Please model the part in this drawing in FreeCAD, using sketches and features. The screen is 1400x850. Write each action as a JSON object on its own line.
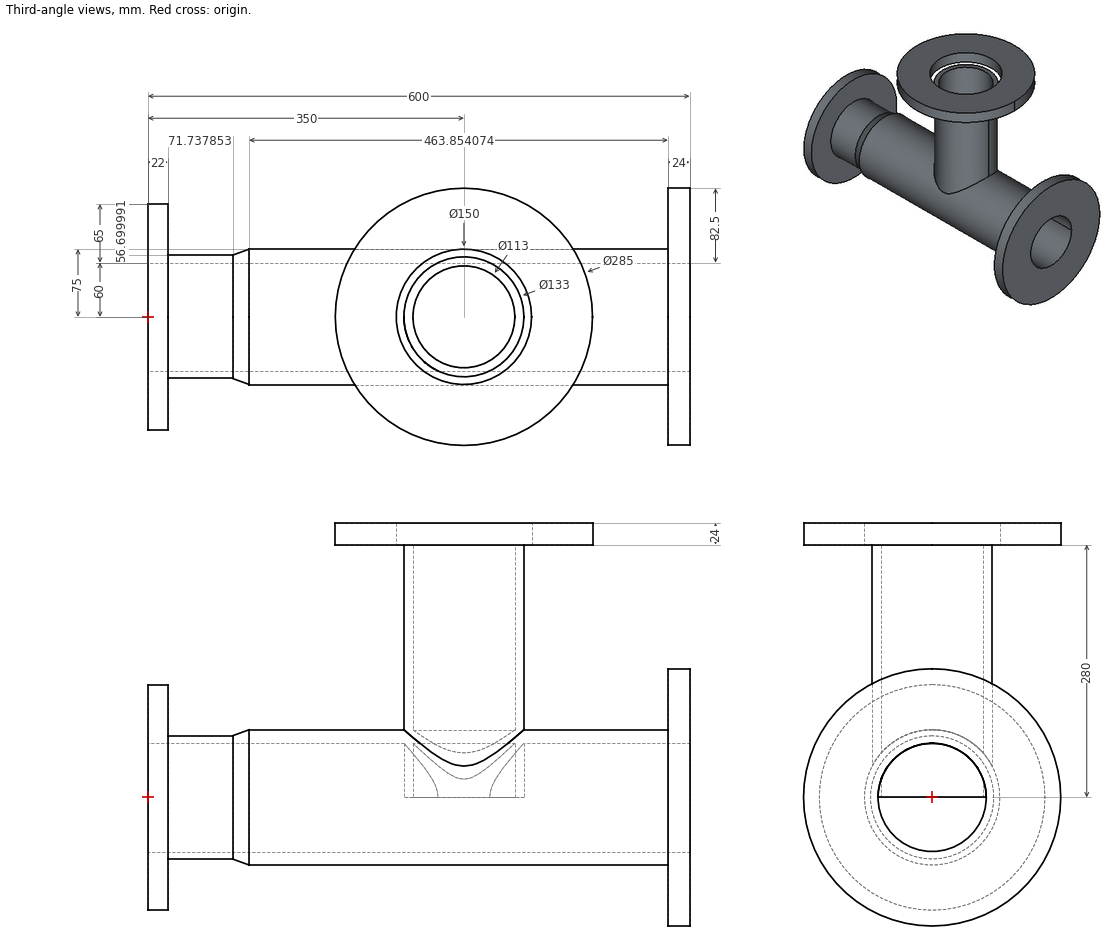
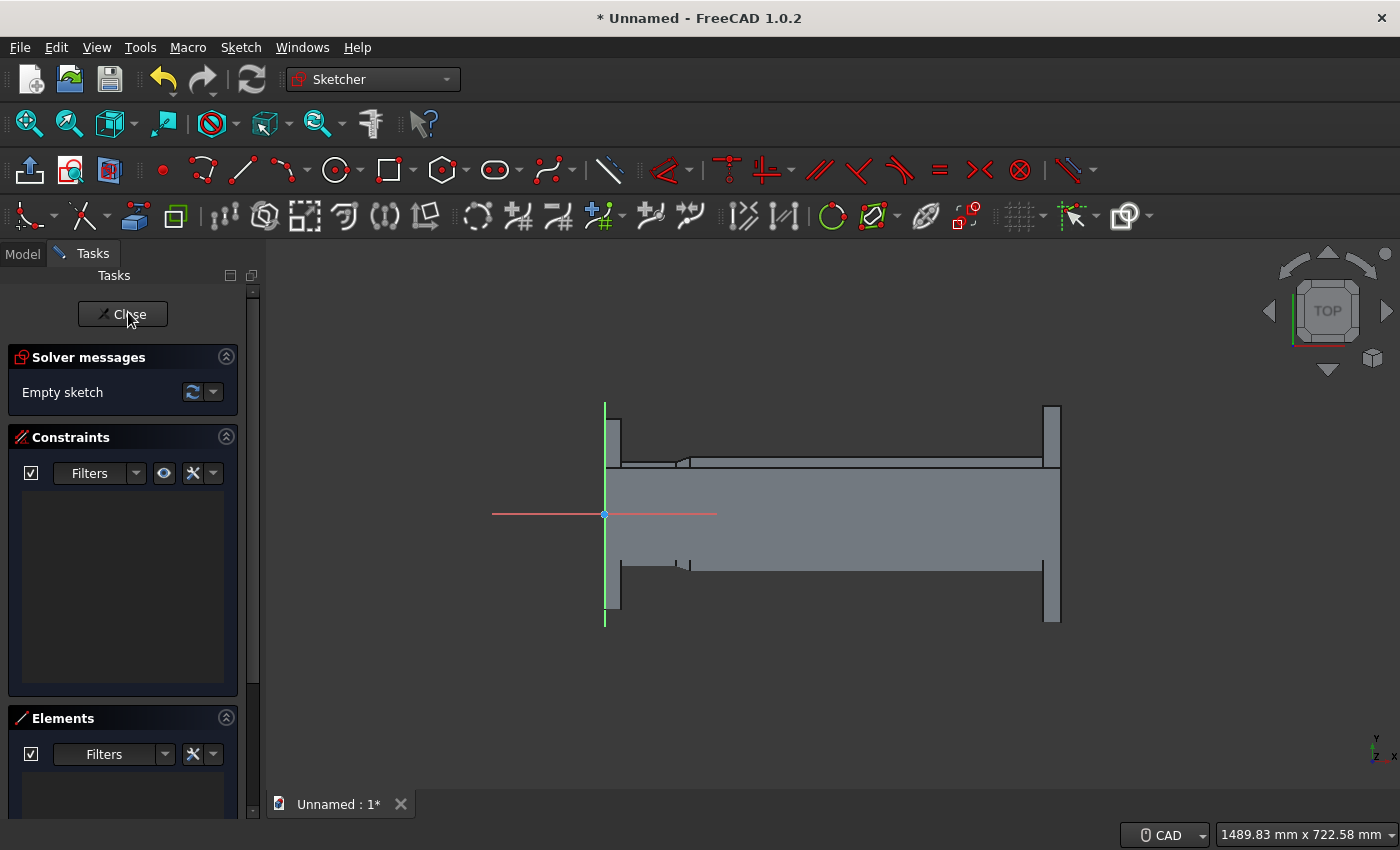
{"action": "scroll", "coordinate": [917, 514], "scroll_direction": "up", "scroll_amount": 6}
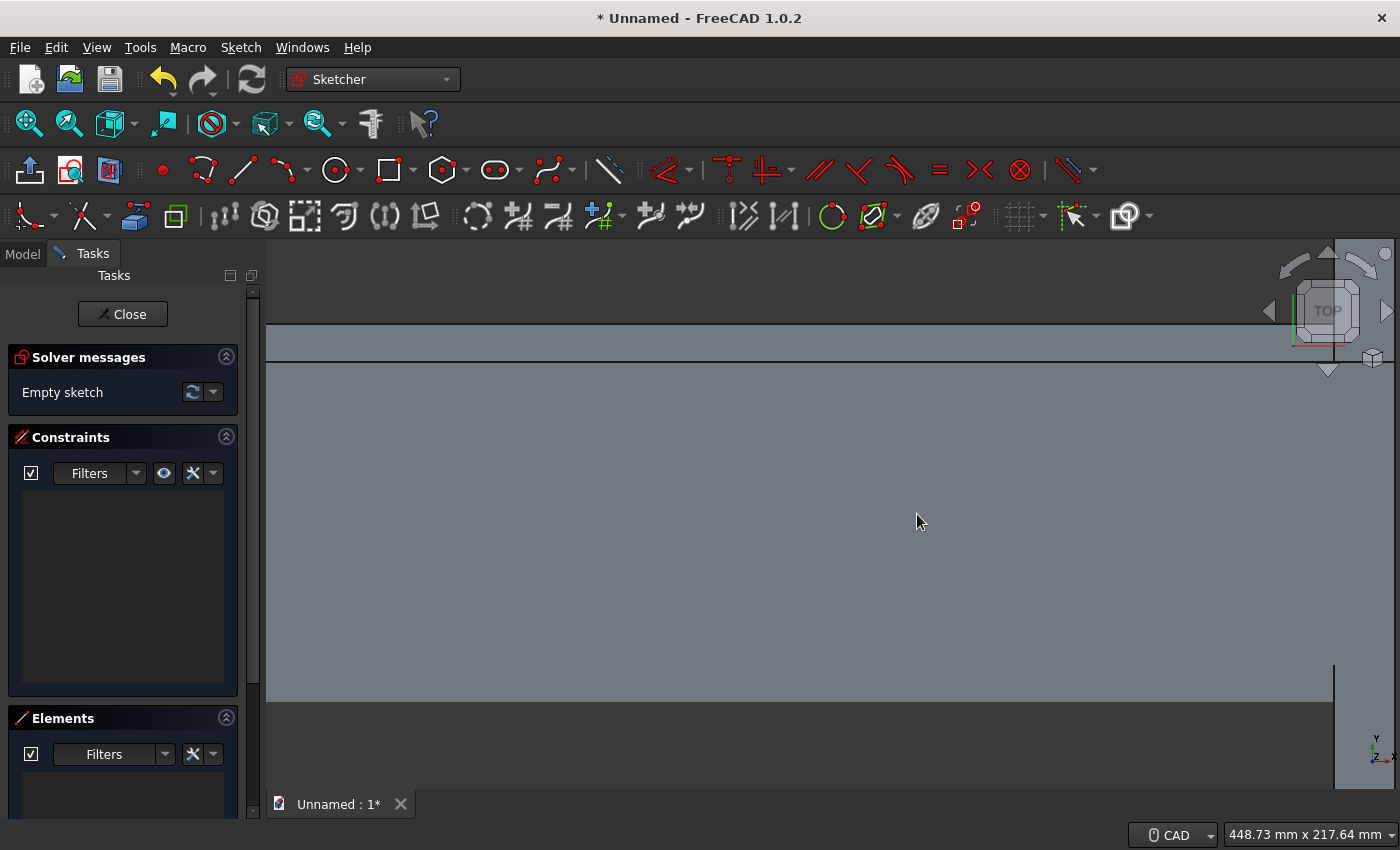
{"action": "key", "text": "g c"}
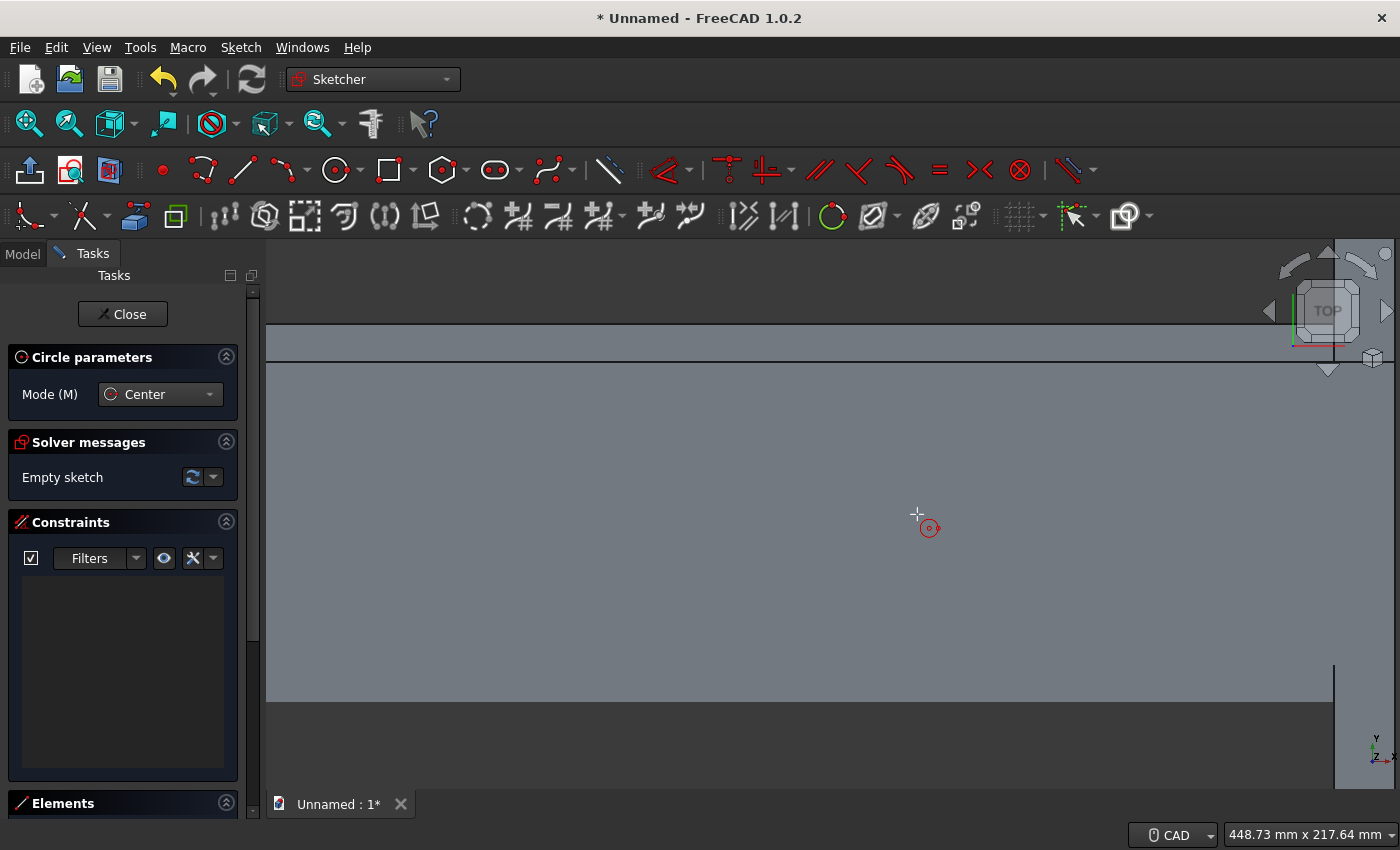
{"action": "left_click", "coordinate": [763, 513]}
{"action": "mouse_move", "coordinate": [882, 394]}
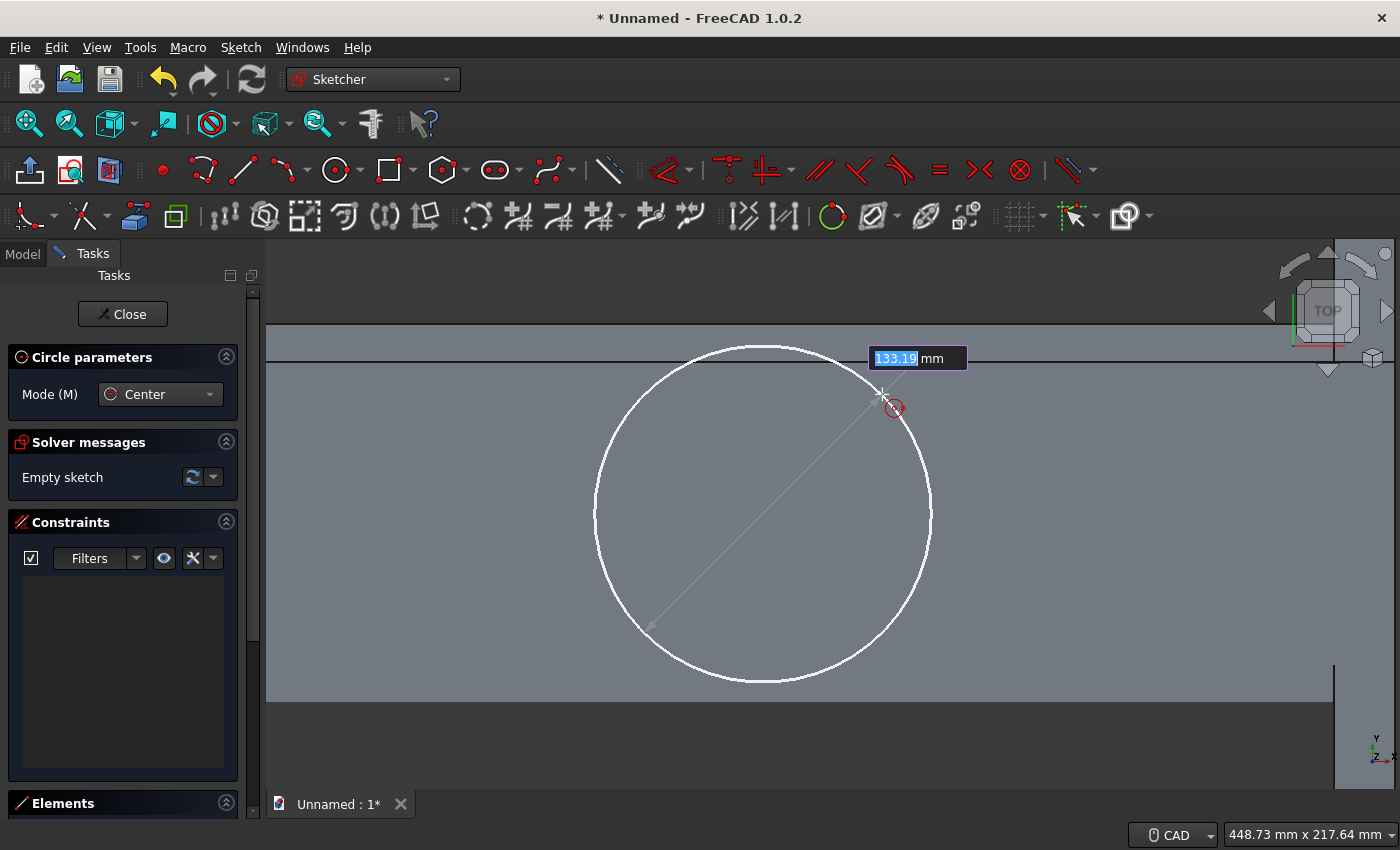
{"action": "type", "text": "133"}
{"action": "key", "text": "Return"}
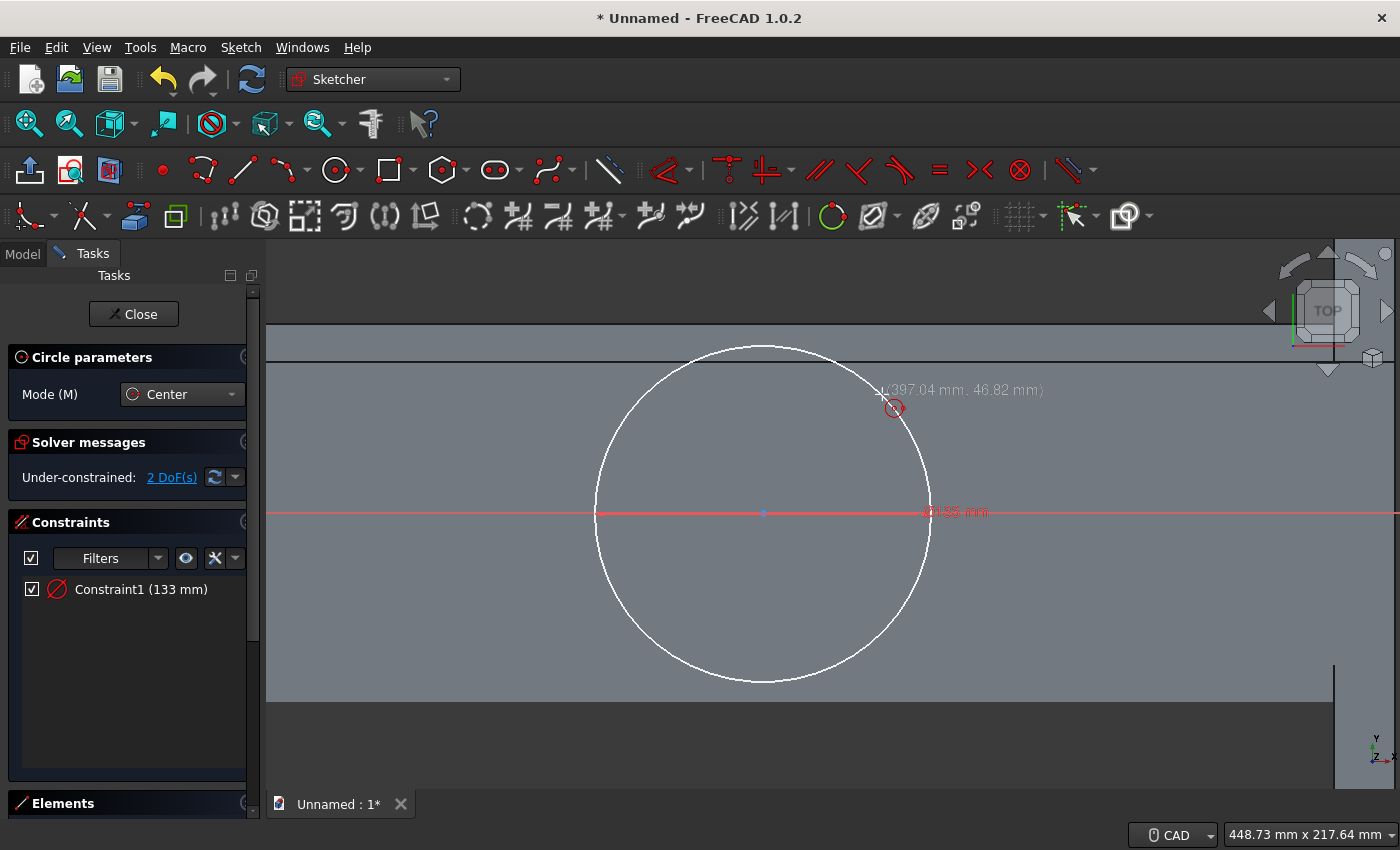
{"action": "left_click", "coordinate": [763, 514]}
{"action": "mouse_move", "coordinate": [864, 412]}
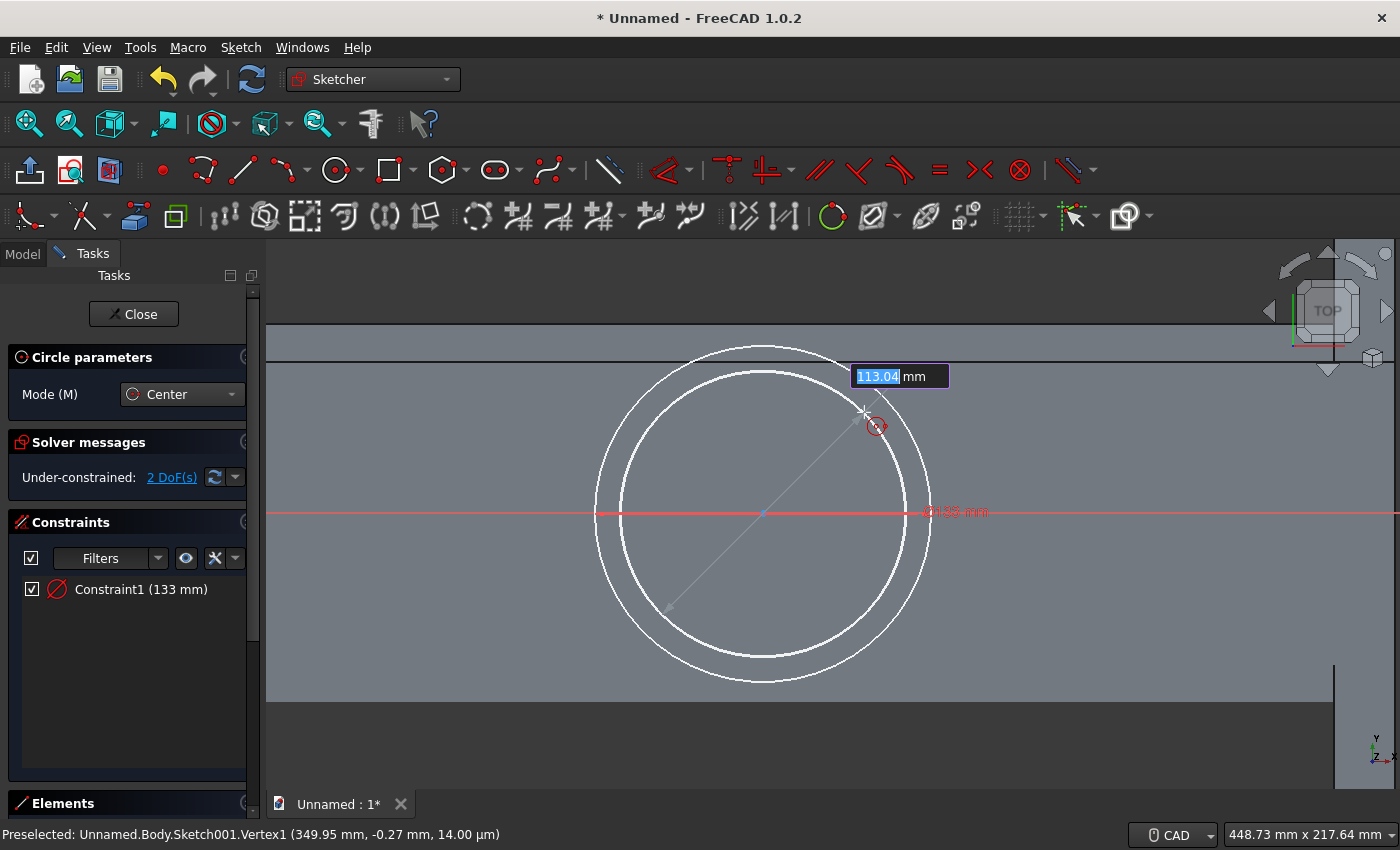
{"action": "type", "text": "113"}
{"action": "key", "text": "Return"}
{"action": "key", "text": "Escape"}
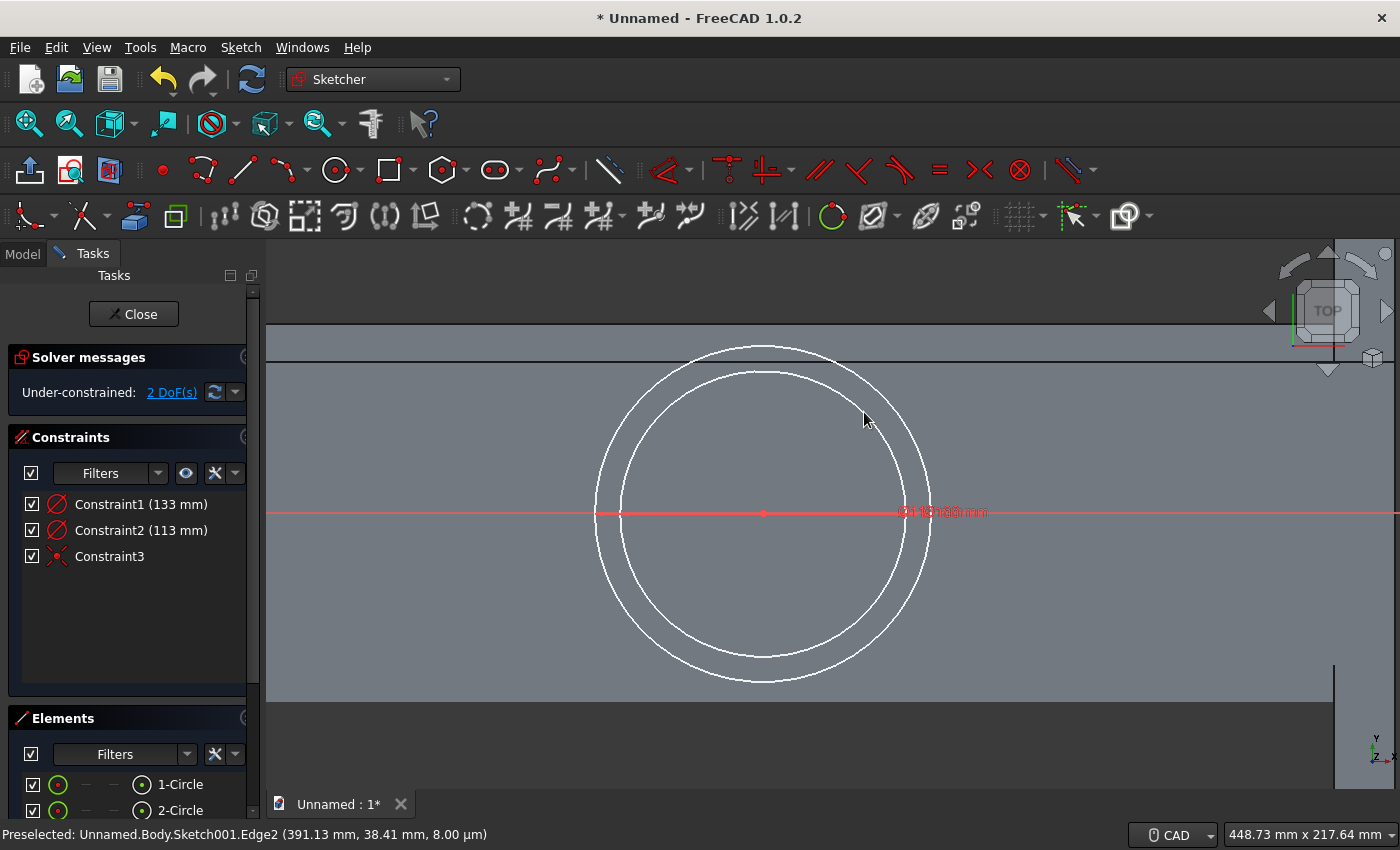
{"action": "left_click", "coordinate": [763, 514]}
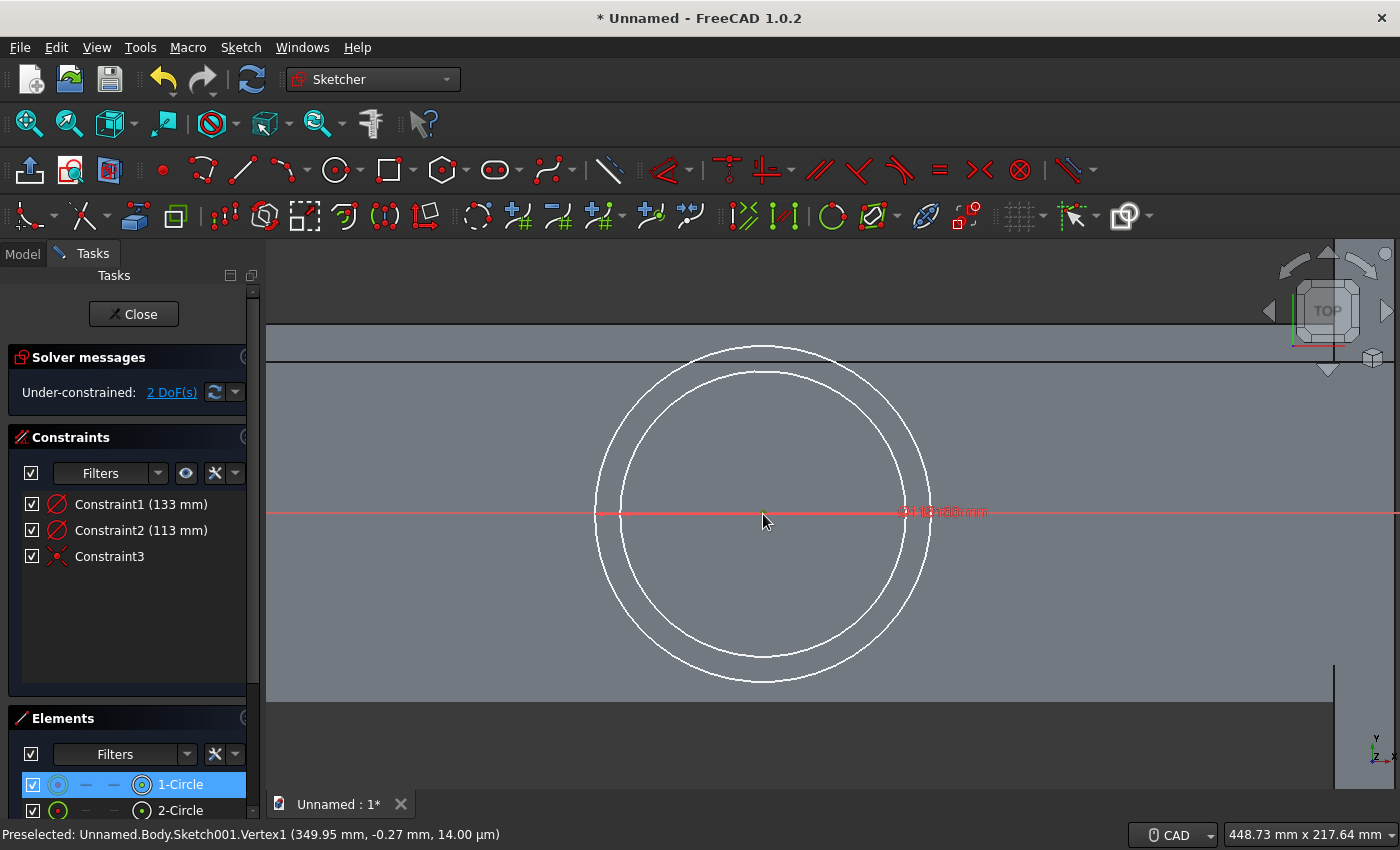
{"action": "left_click", "coordinate": [361, 513]}